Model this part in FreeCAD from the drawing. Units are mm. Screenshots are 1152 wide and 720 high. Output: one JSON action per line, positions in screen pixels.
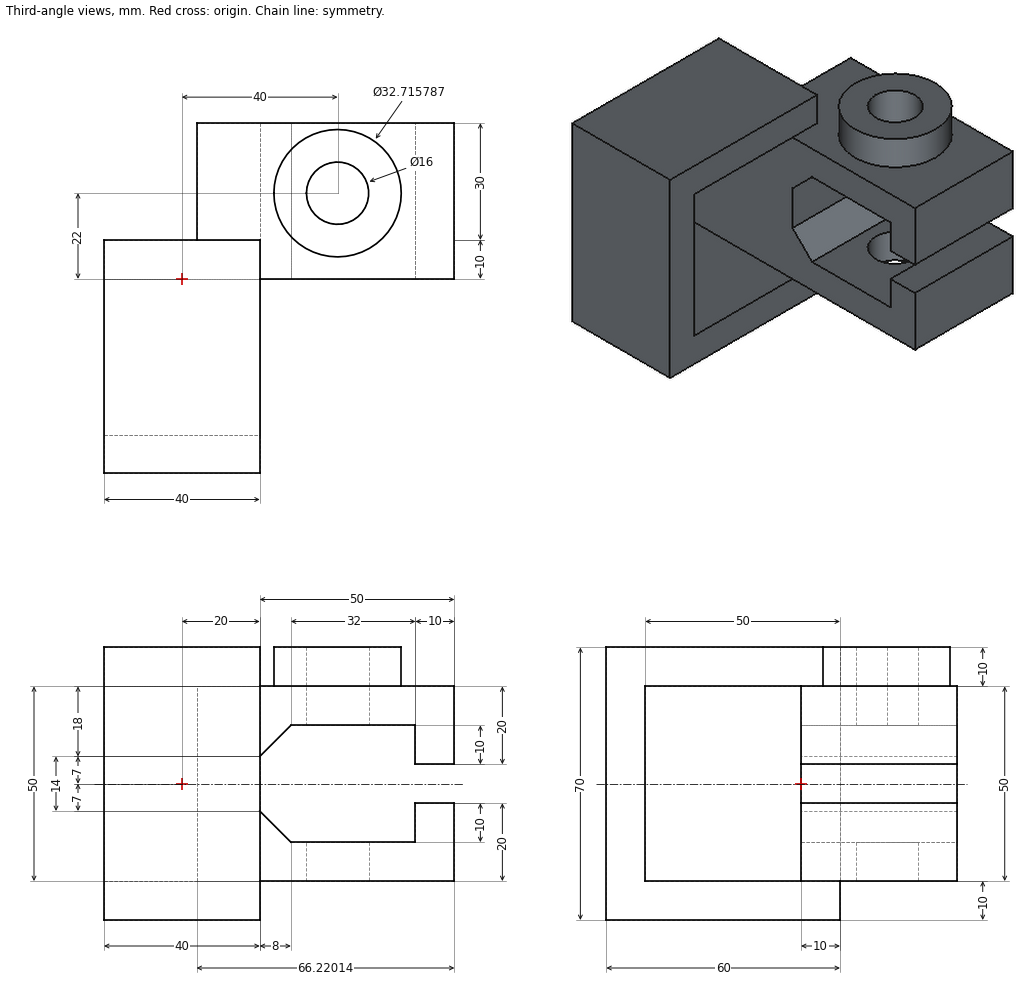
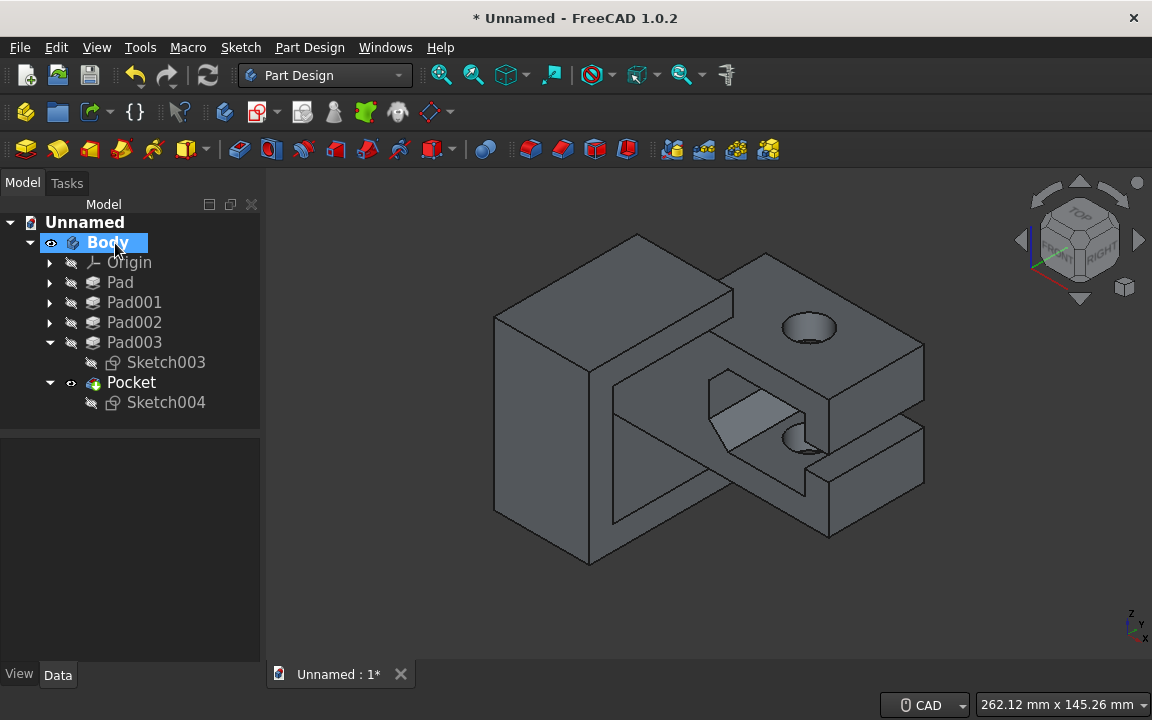
{"action": "left_click", "coordinate": [766, 291]}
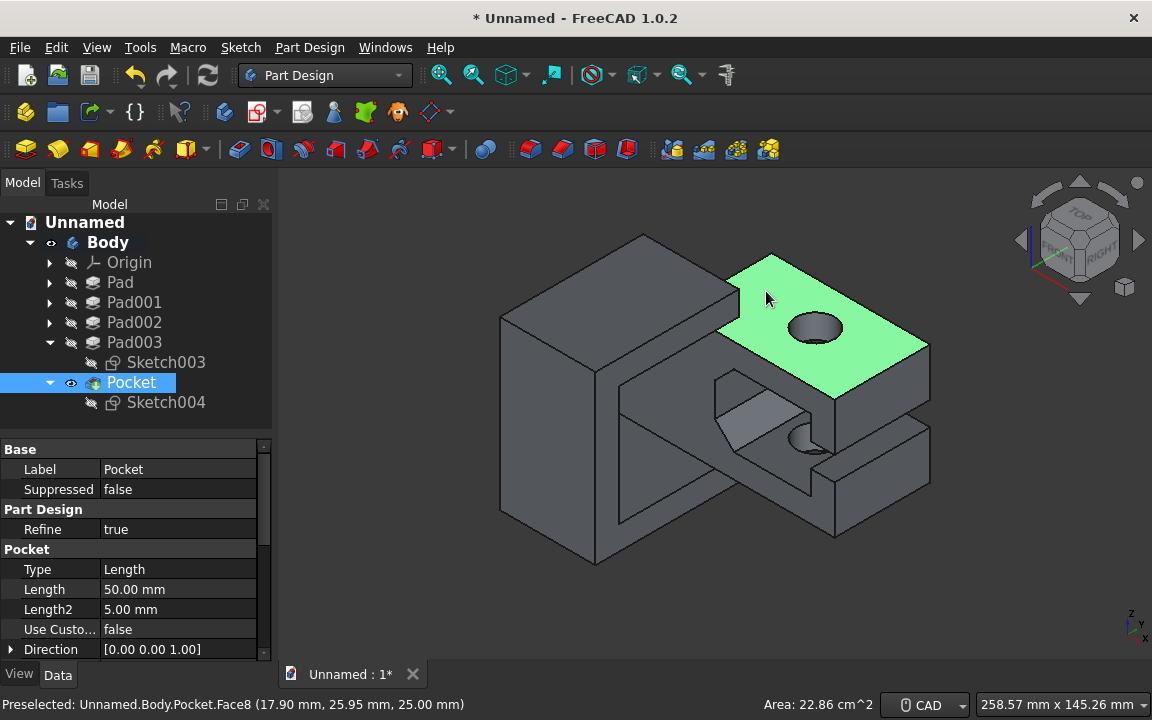
{"action": "left_click", "coordinate": [258, 112]}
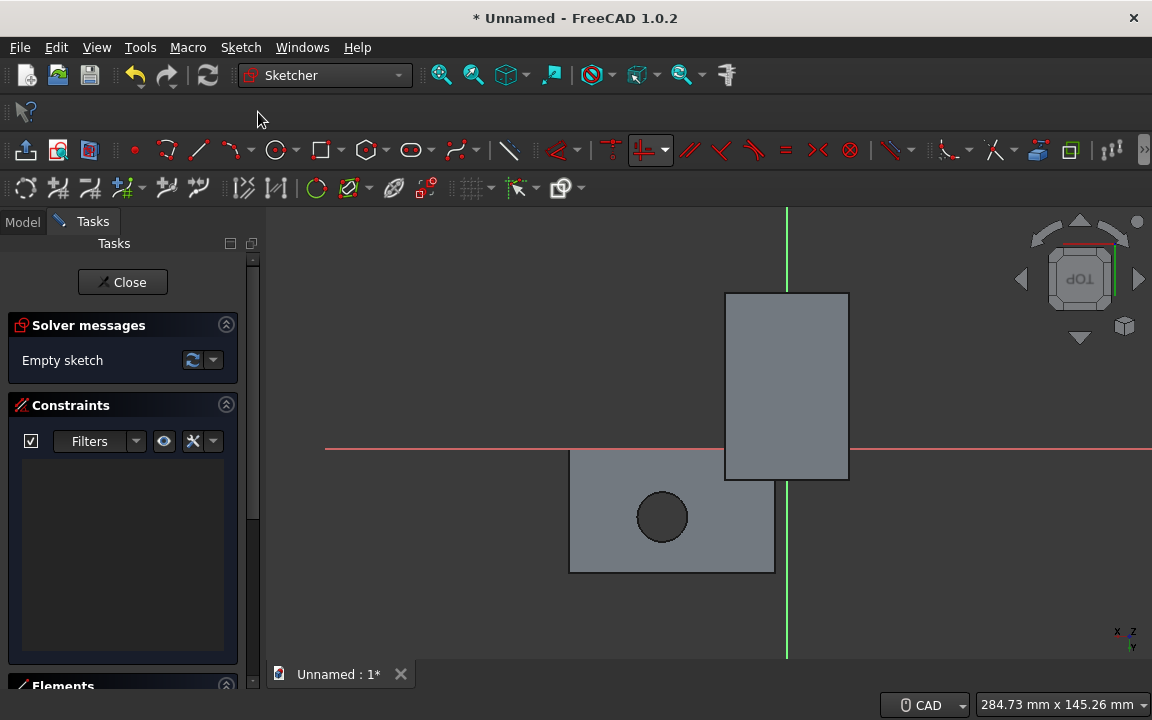
{"action": "key", "text": "q s"}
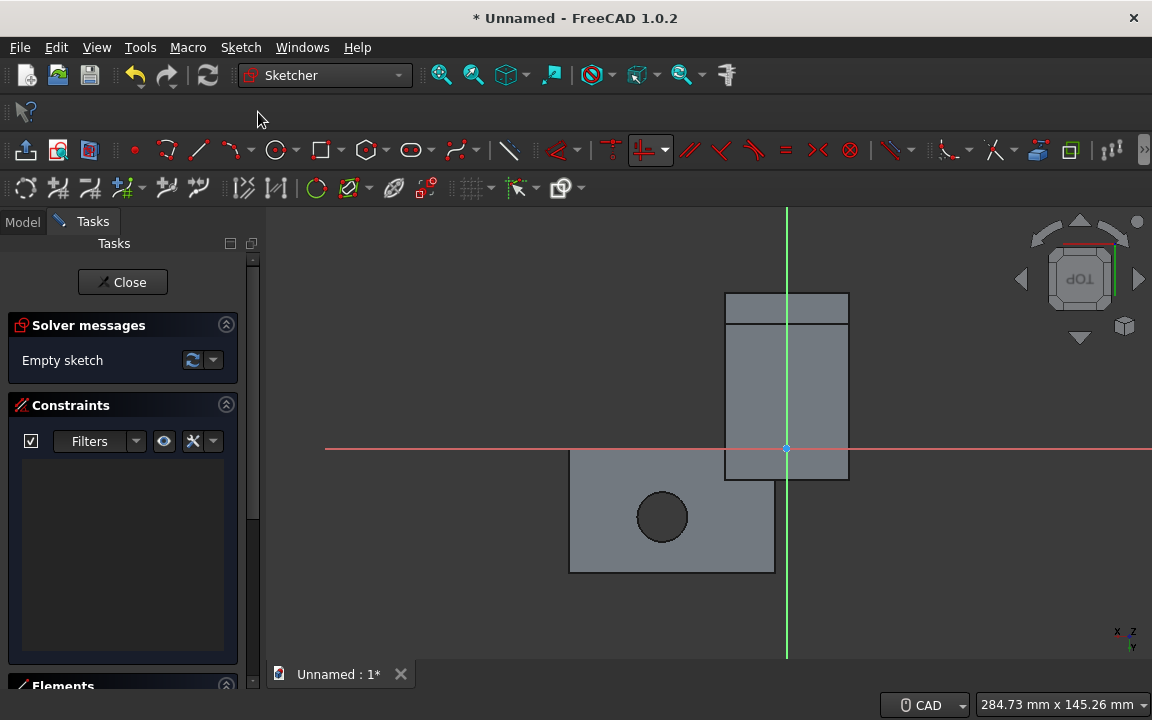
{"action": "scroll", "coordinate": [747, 570], "scroll_direction": "up", "scroll_amount": 4}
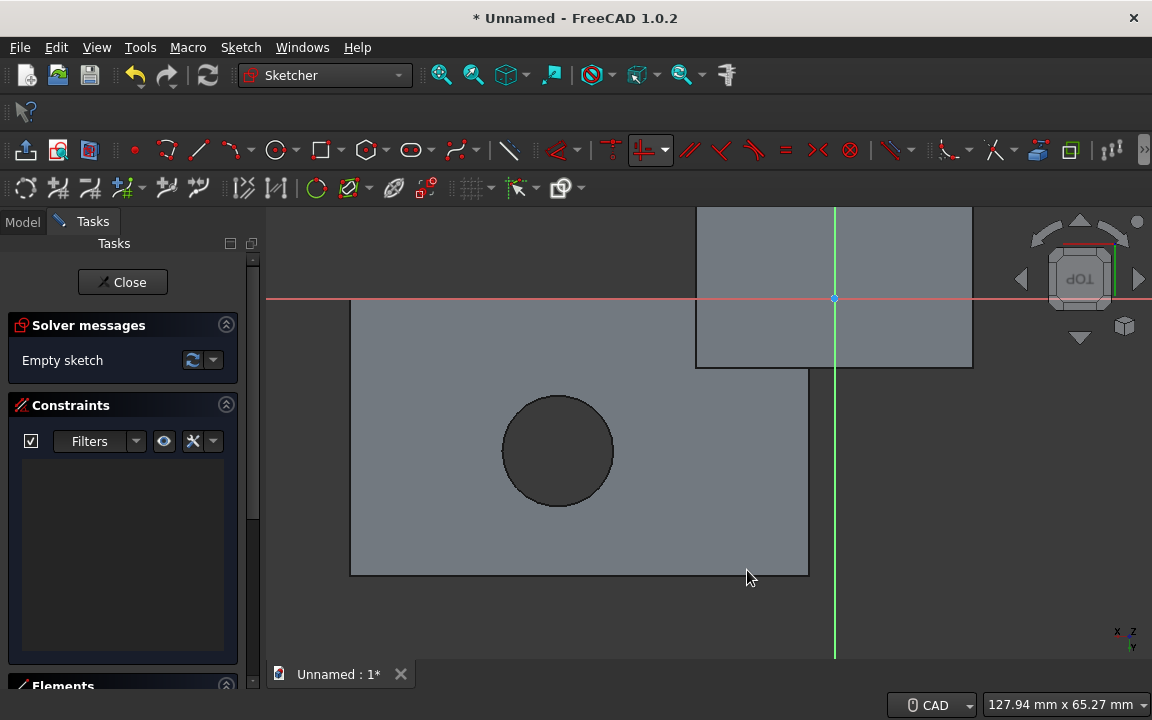
{"action": "key", "text": "g c"}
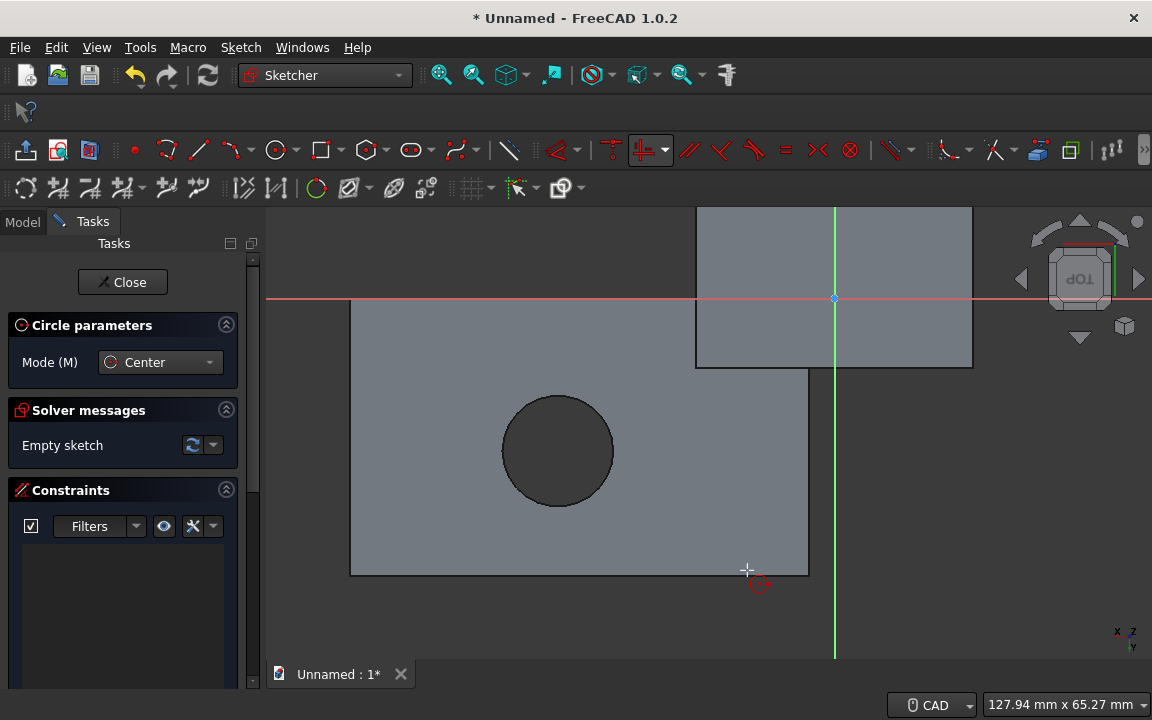
{"action": "left_click", "coordinate": [558, 451]}
{"action": "left_click", "coordinate": [638, 371]}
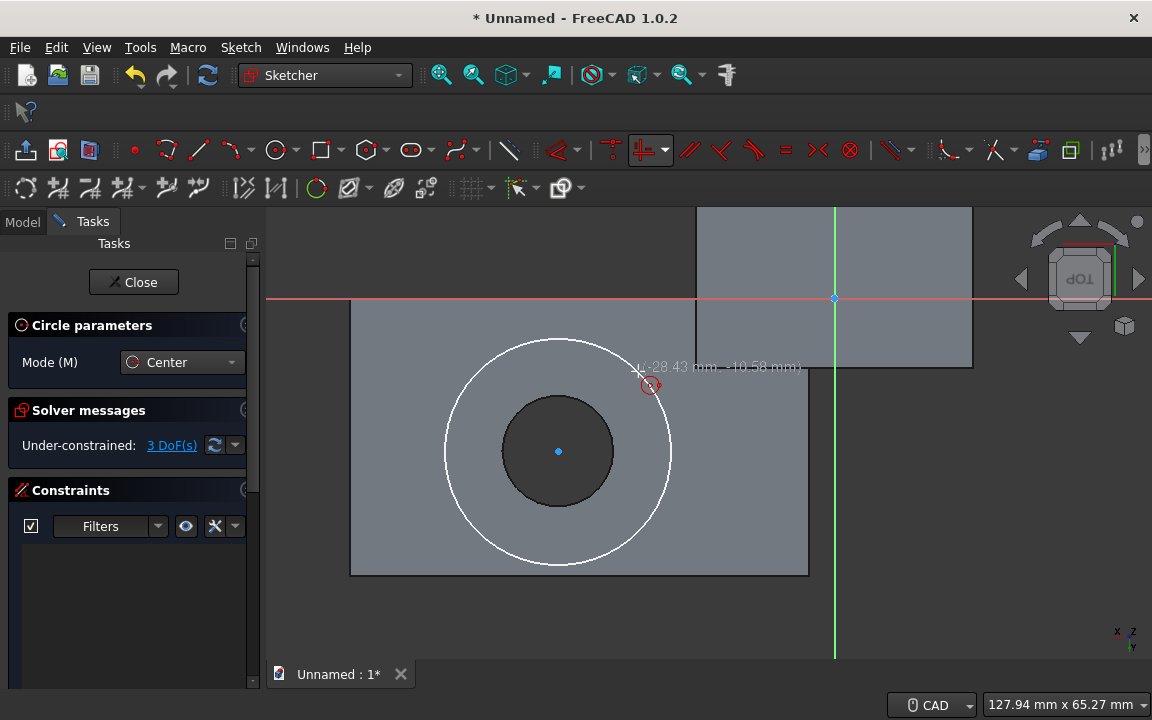
{"action": "left_click", "coordinate": [558, 452]}
{"action": "left_click", "coordinate": [597, 412]}
{"action": "key", "text": "Escape"}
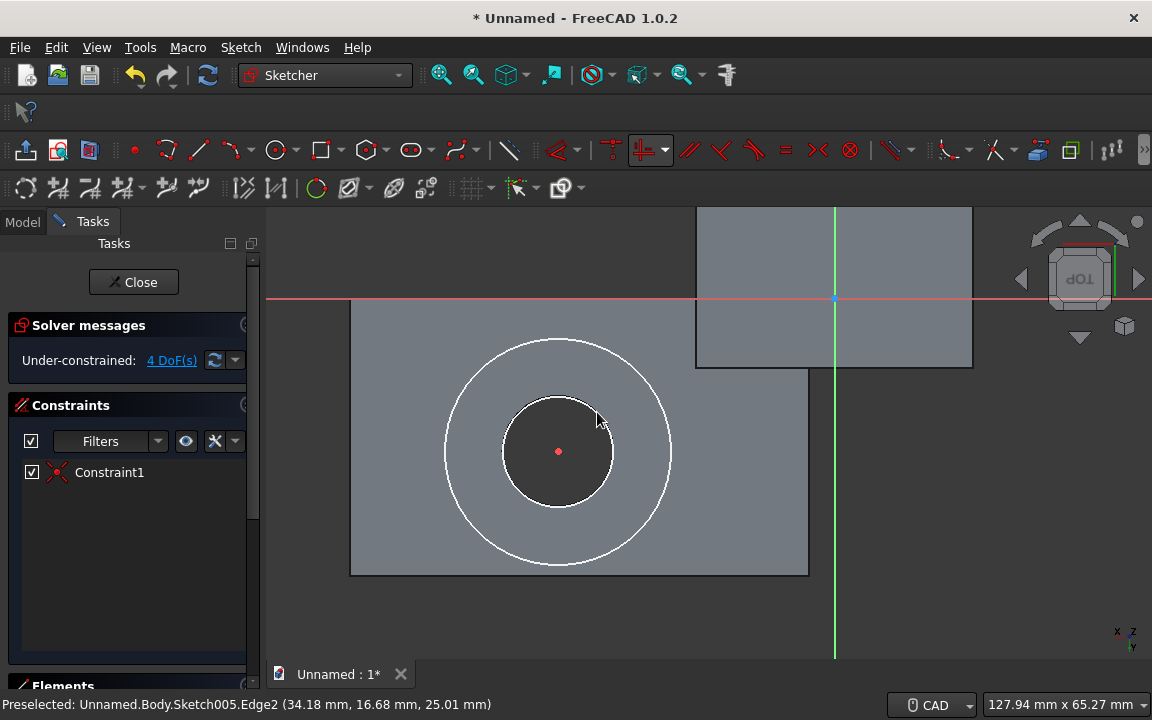
{"action": "left_click", "coordinate": [556, 150]}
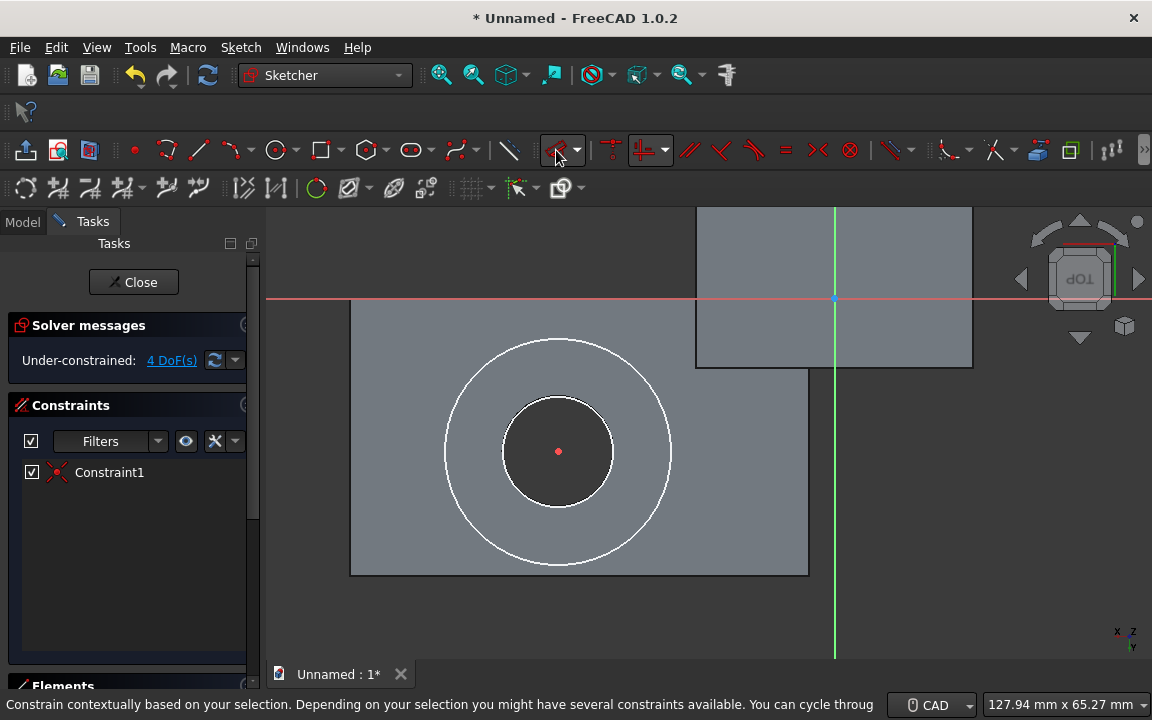
{"action": "left_click", "coordinate": [638, 372]}
{"action": "left_click", "coordinate": [661, 349]}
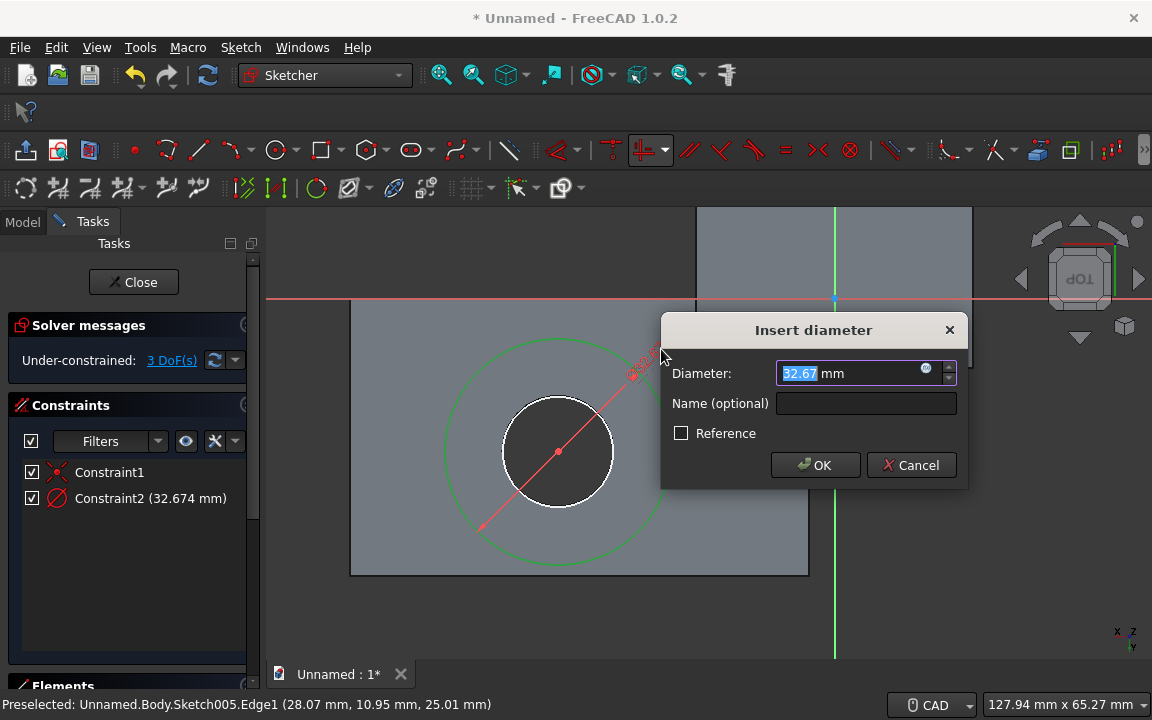
{"action": "type", "text": "32.715787"}
{"action": "key", "text": "Return"}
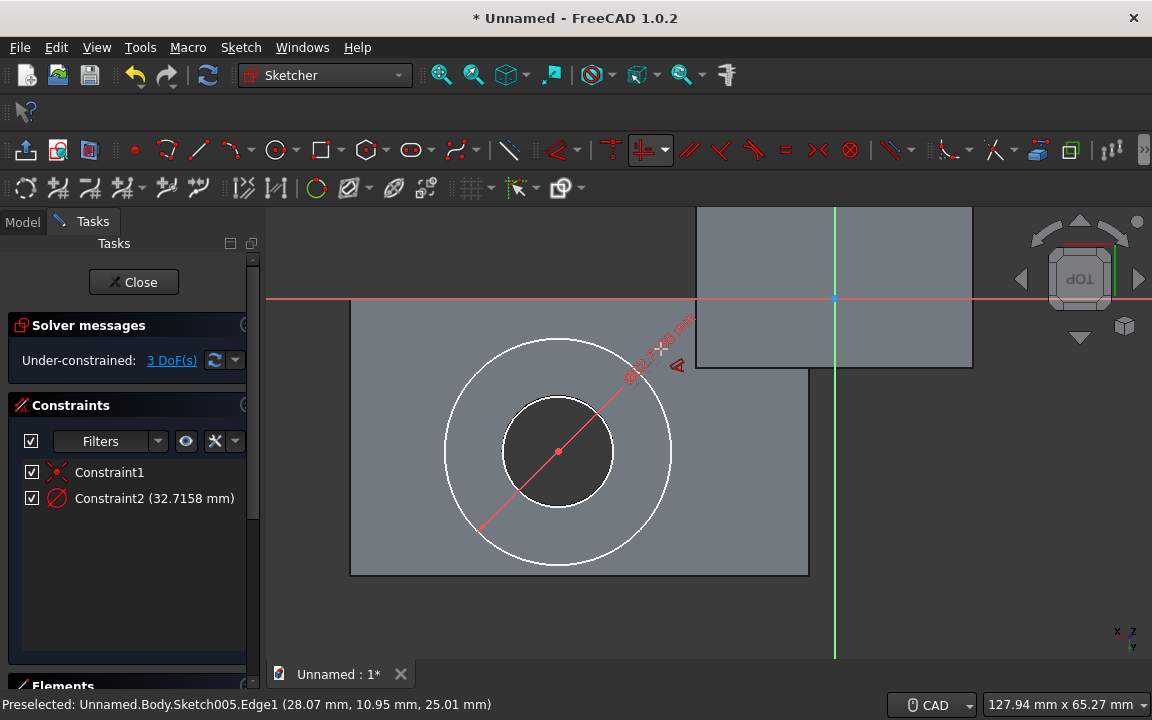
{"action": "left_click", "coordinate": [597, 413]}
{"action": "left_click", "coordinate": [620, 390]}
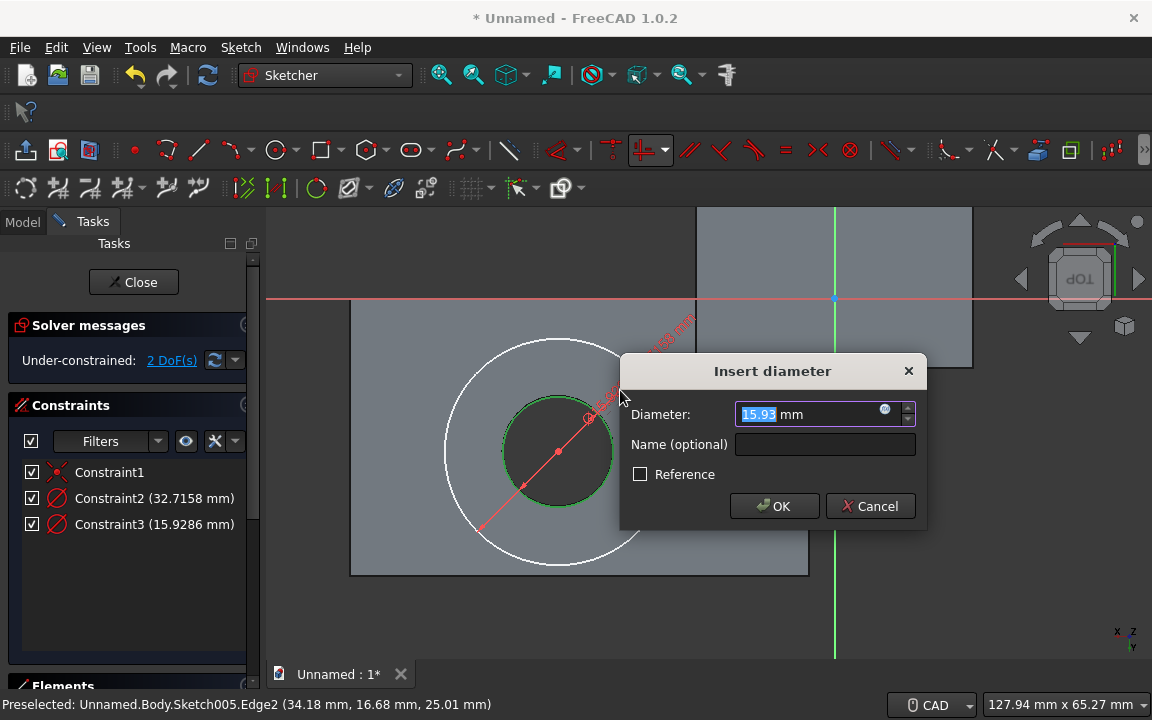
{"action": "type", "text": "16"}
{"action": "key", "text": "Return"}